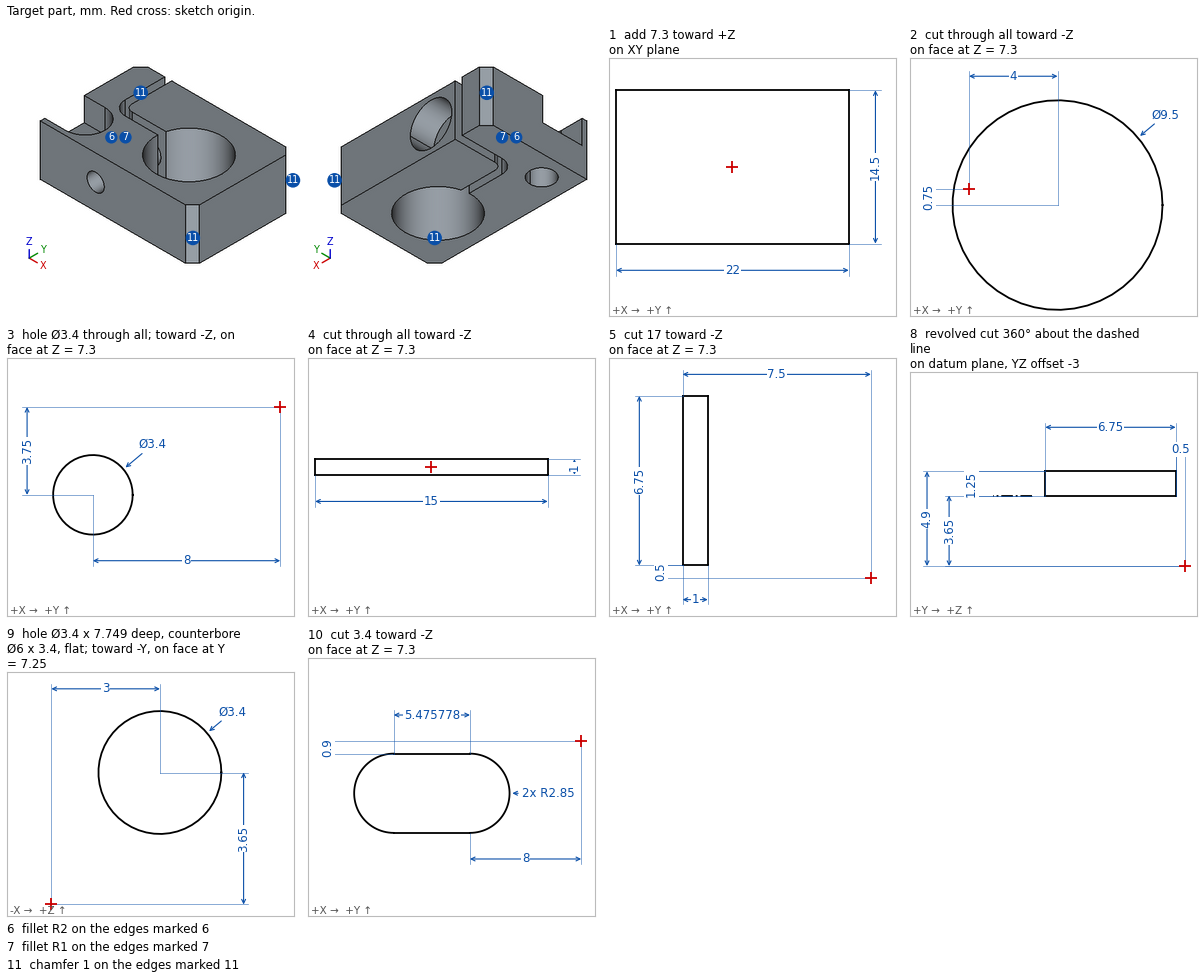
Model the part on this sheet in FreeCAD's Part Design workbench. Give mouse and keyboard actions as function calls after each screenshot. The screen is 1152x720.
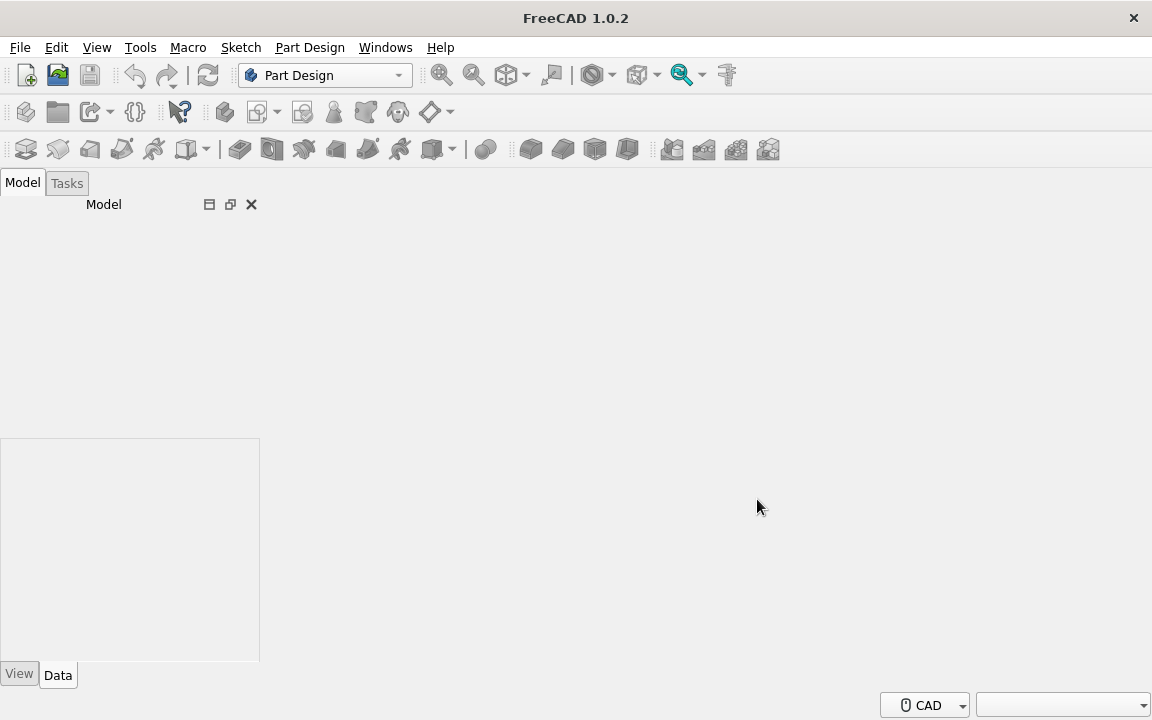
click(26, 76)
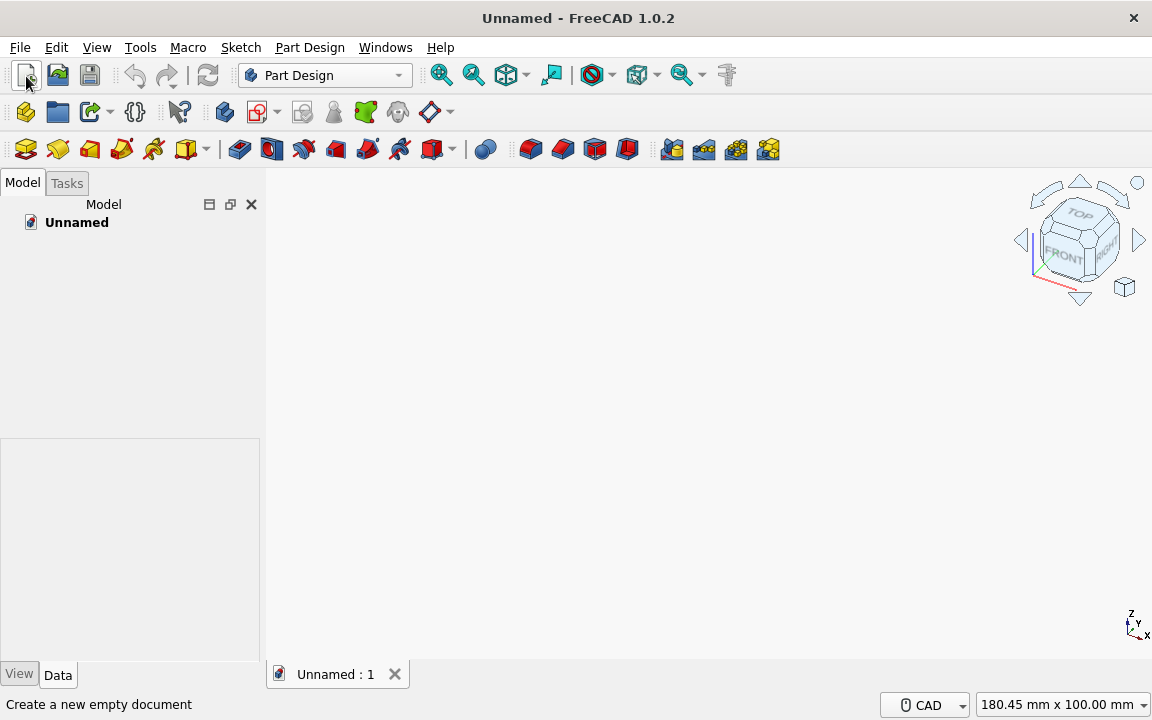
click(258, 112)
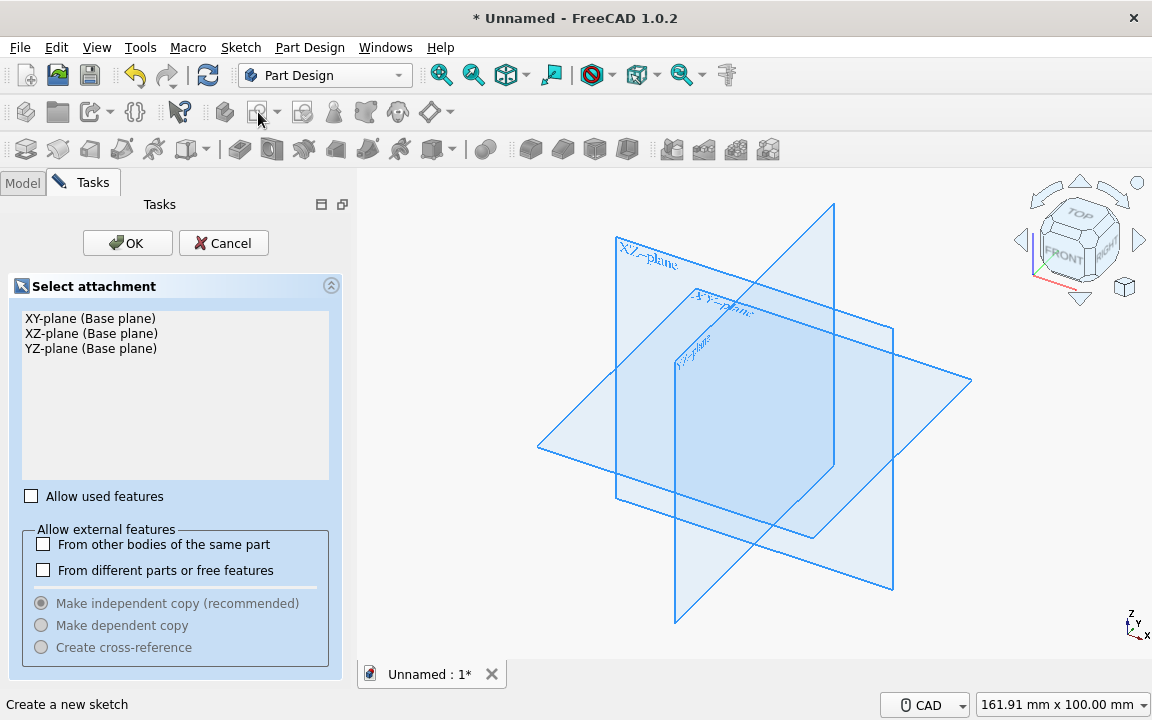
click(82, 318)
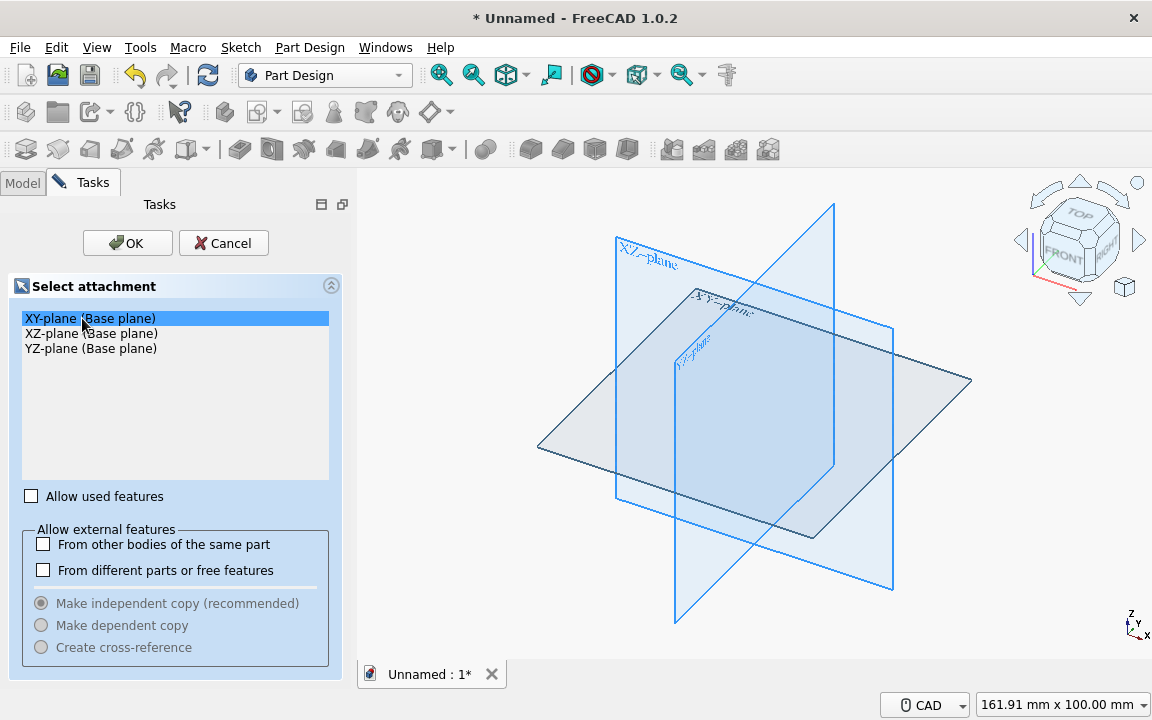
click(128, 243)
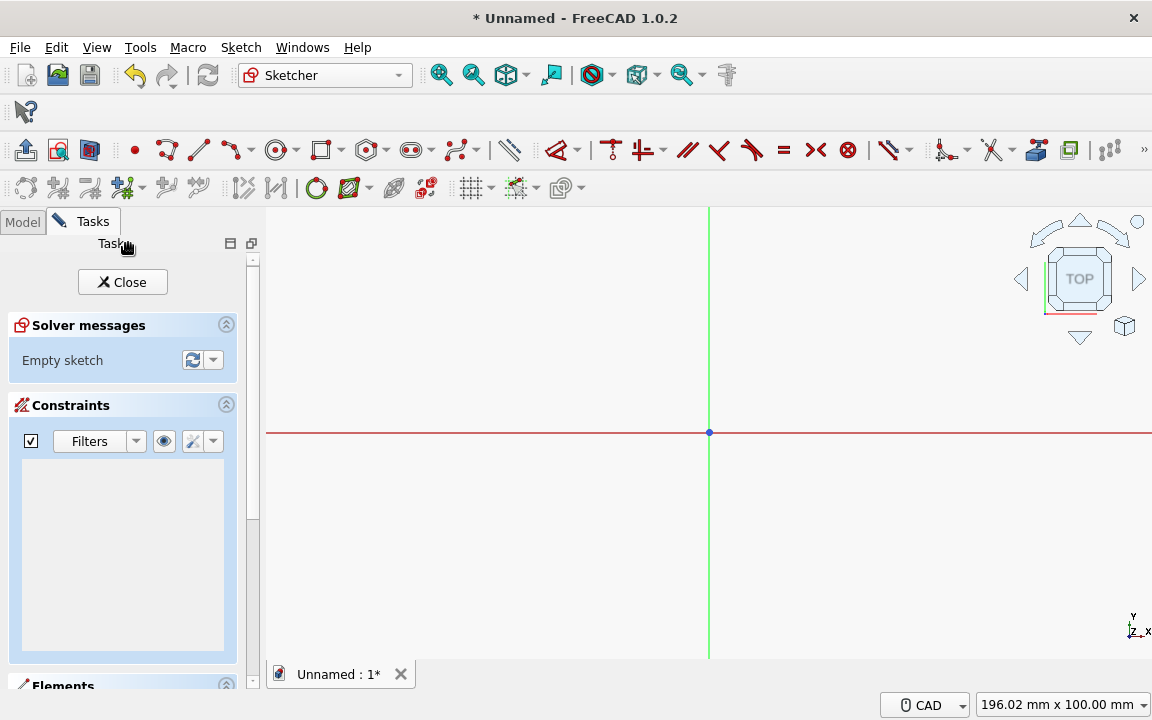
scroll(731, 433, up, 7)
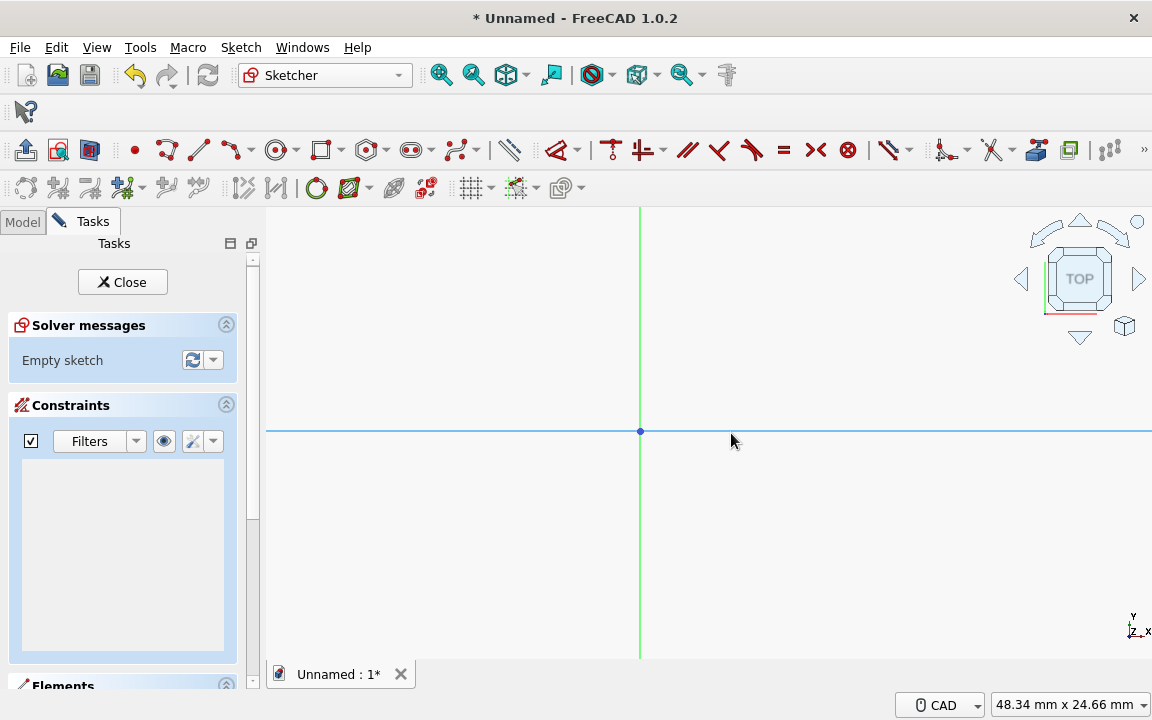
key(g)
key(v)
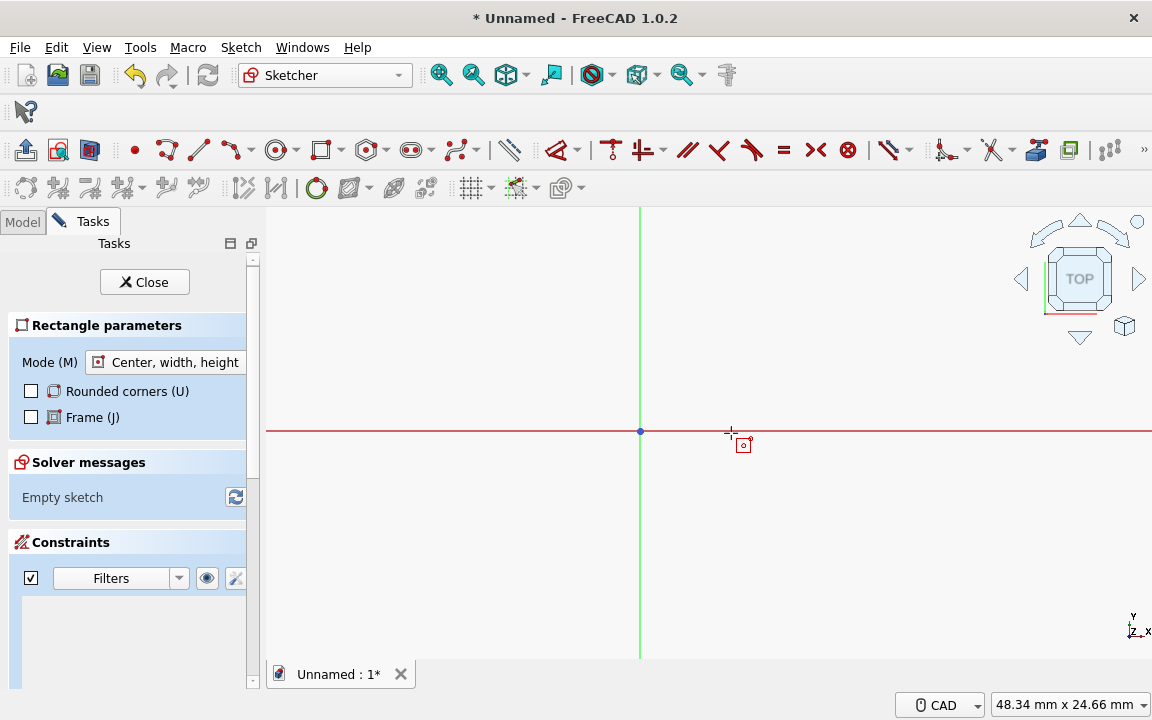
click(640, 431)
click(842, 299)
key(Escape)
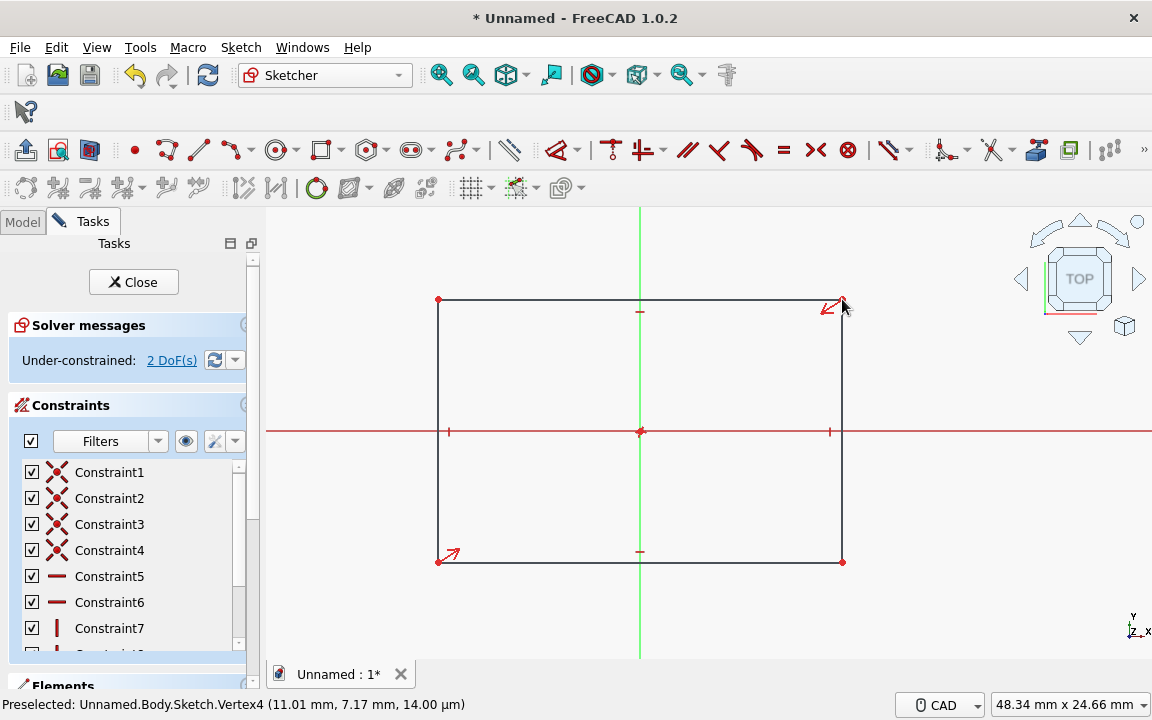
click(556, 150)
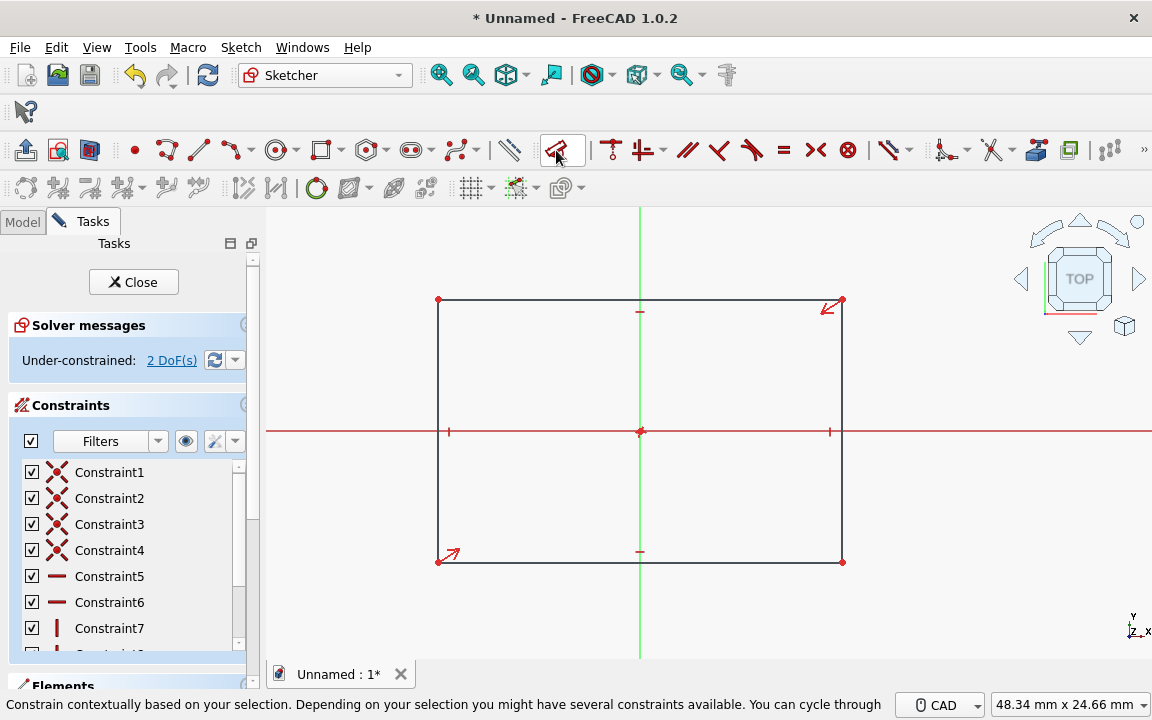
click(559, 563)
click(547, 597)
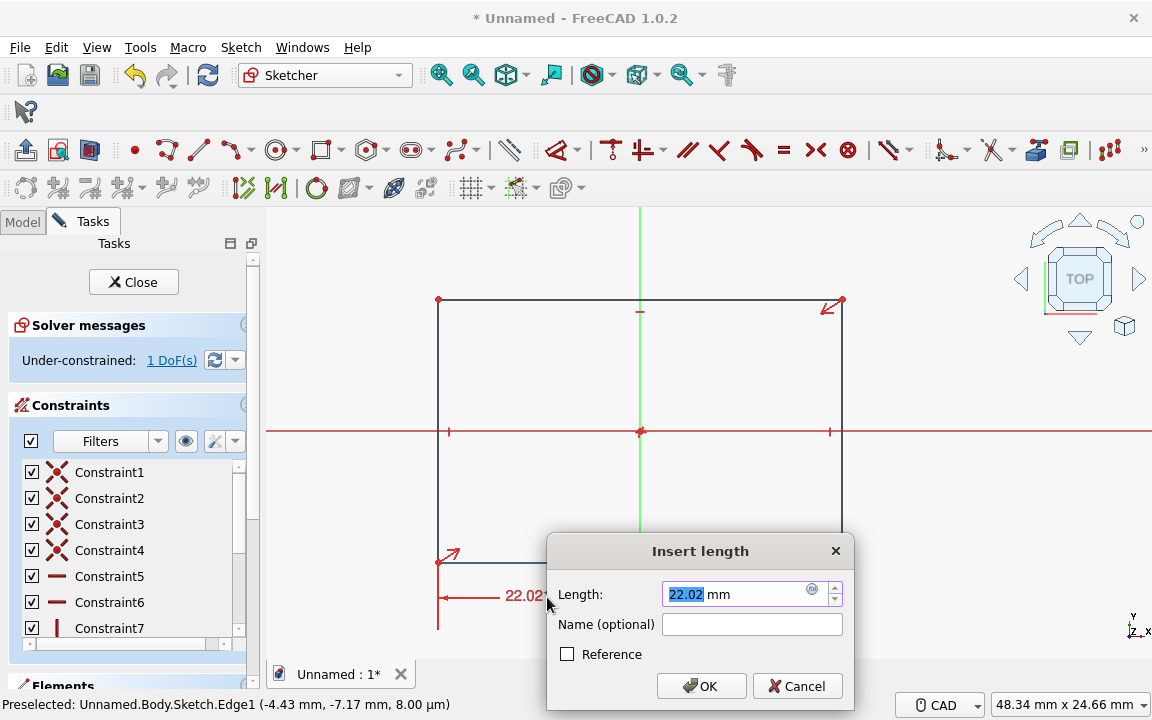
text(22)
key(Return)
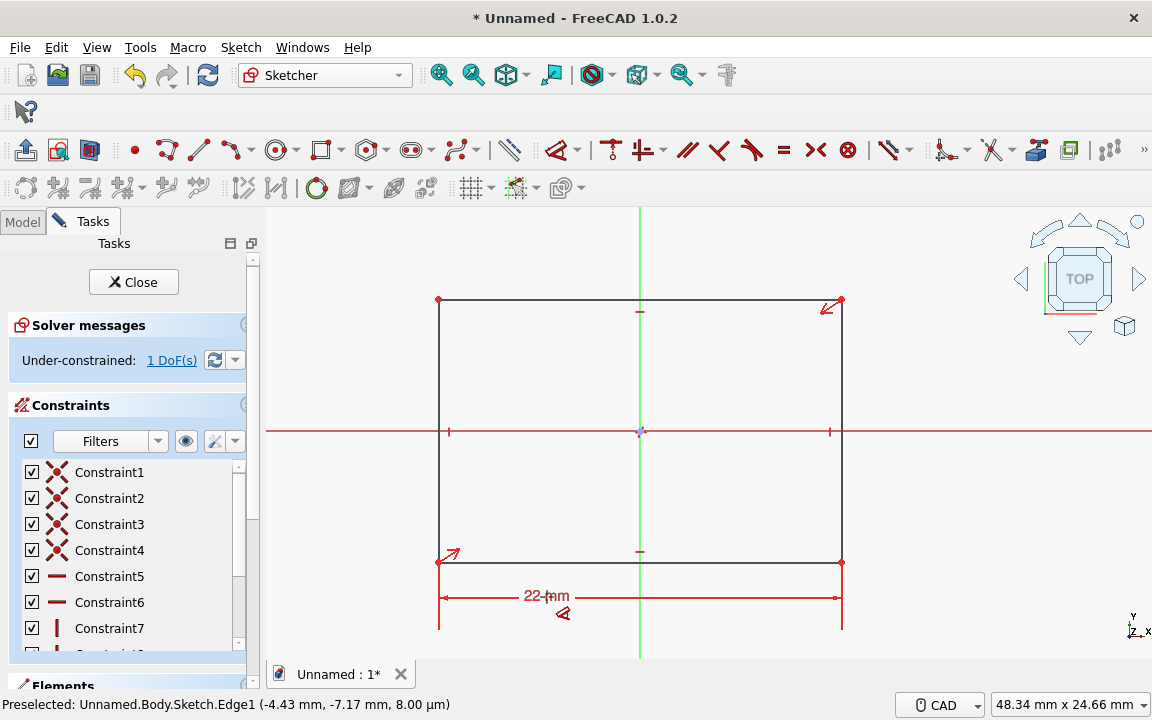
click(842, 484)
click(876, 371)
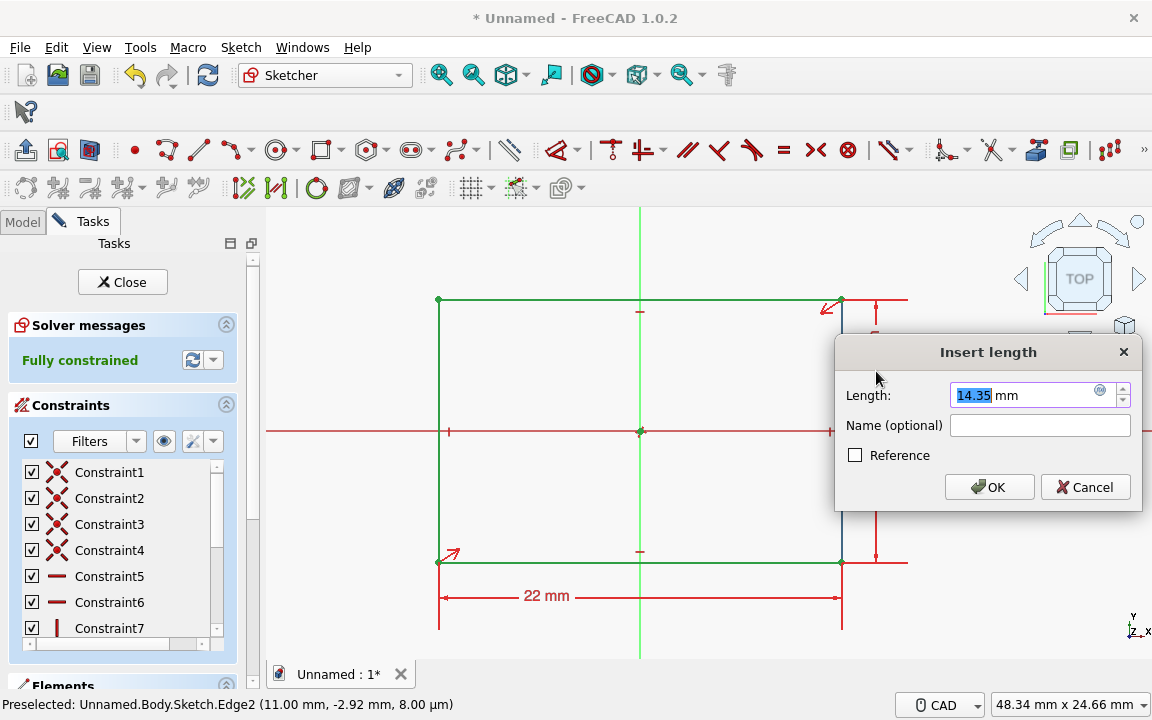
text(14.5)
key(Return)
key(Escape)